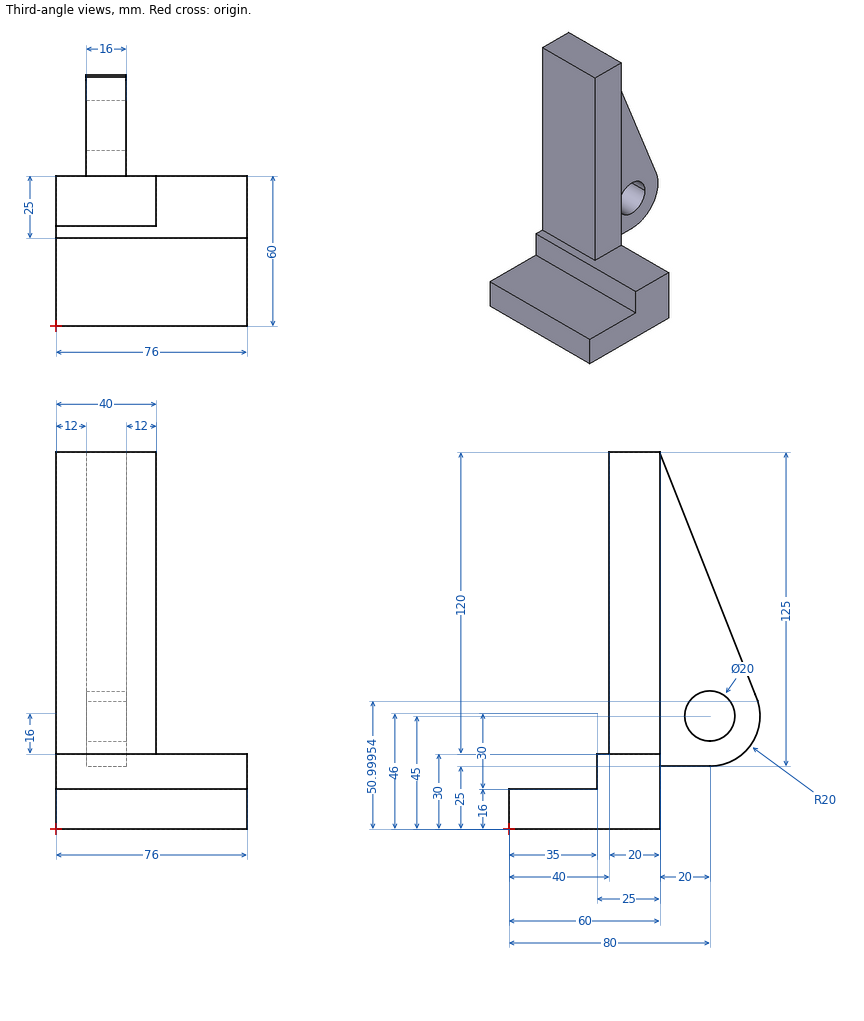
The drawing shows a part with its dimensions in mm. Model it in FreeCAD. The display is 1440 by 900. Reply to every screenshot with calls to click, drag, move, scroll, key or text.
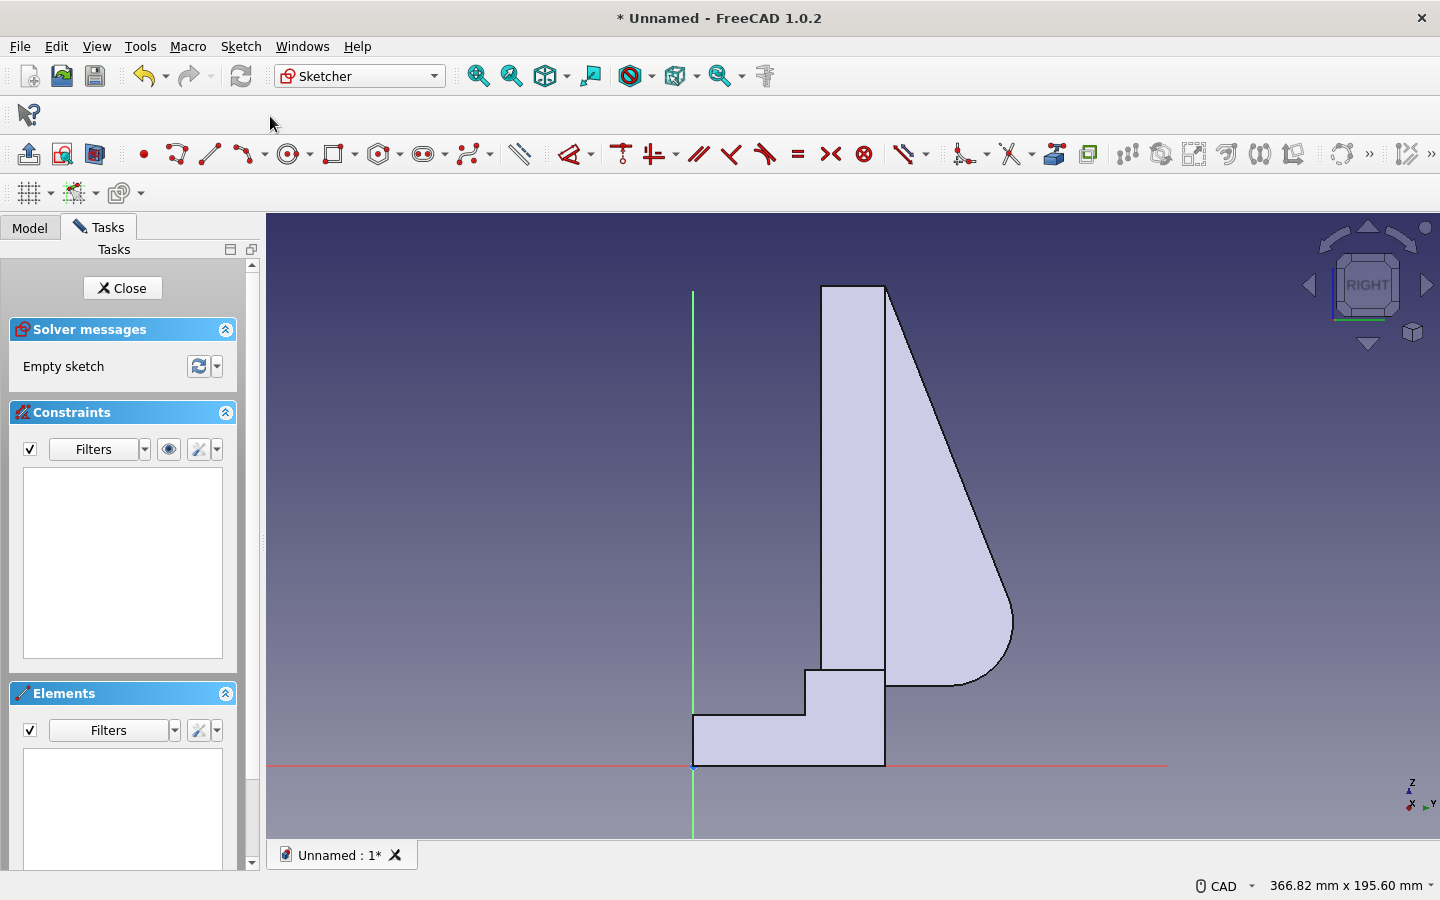
scroll(982, 641, up, 9)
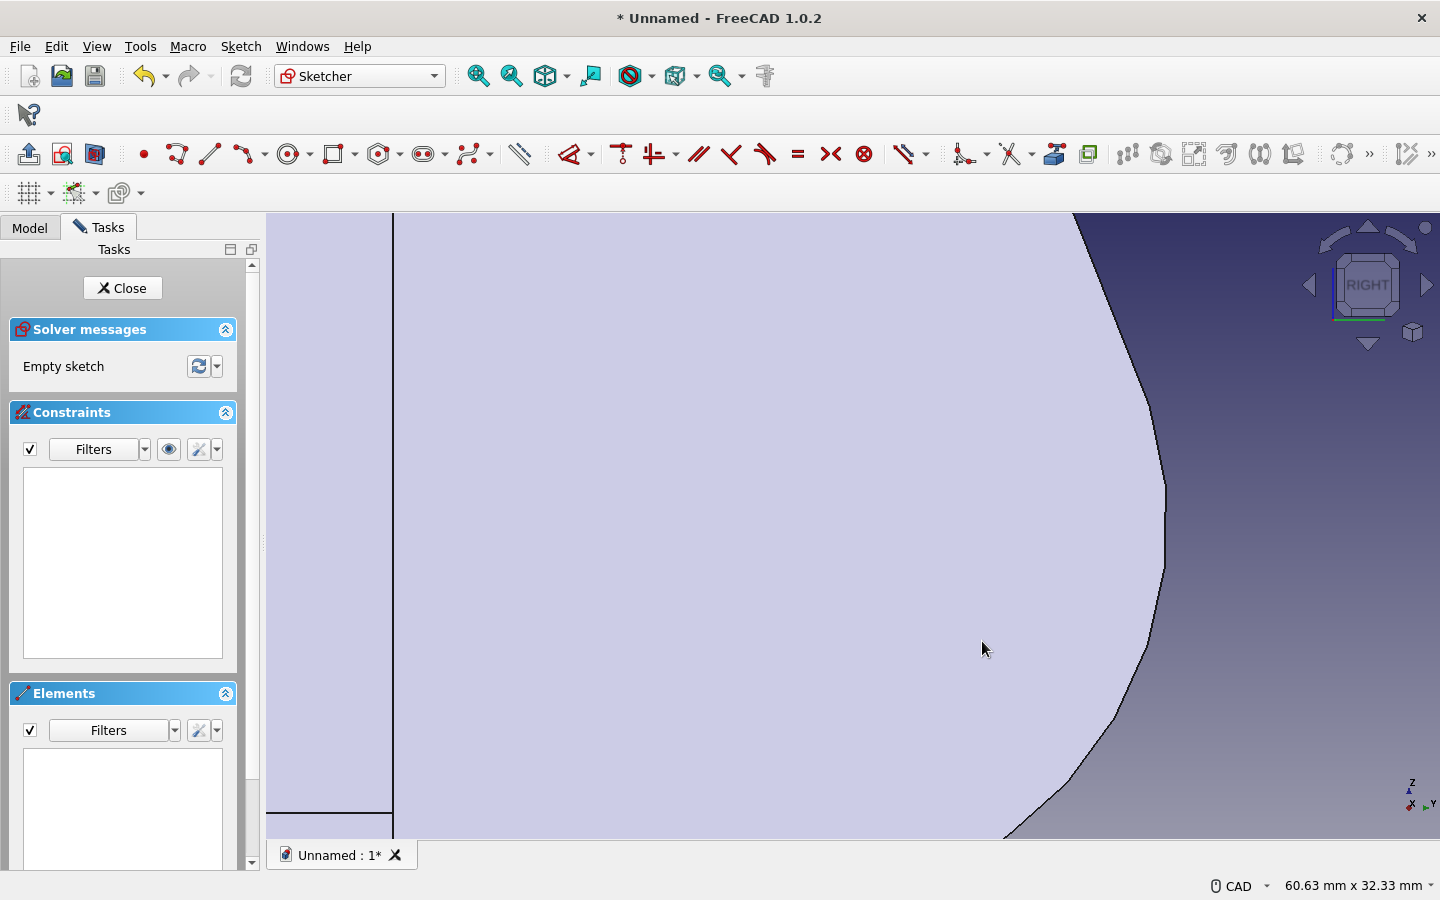
key(g)
key(c)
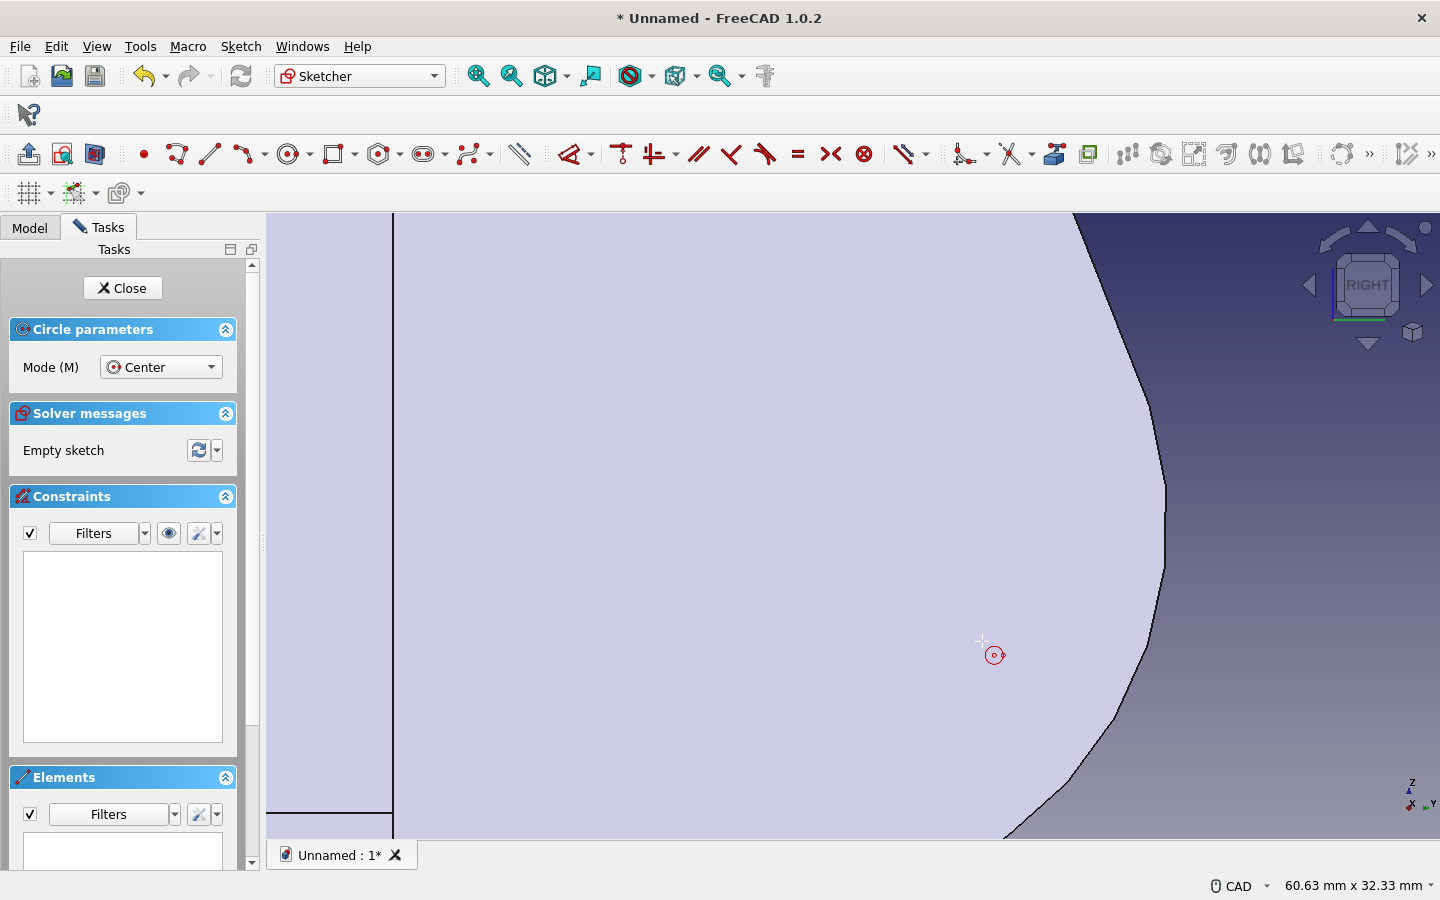
click(780, 523)
click(917, 386)
key(Escape)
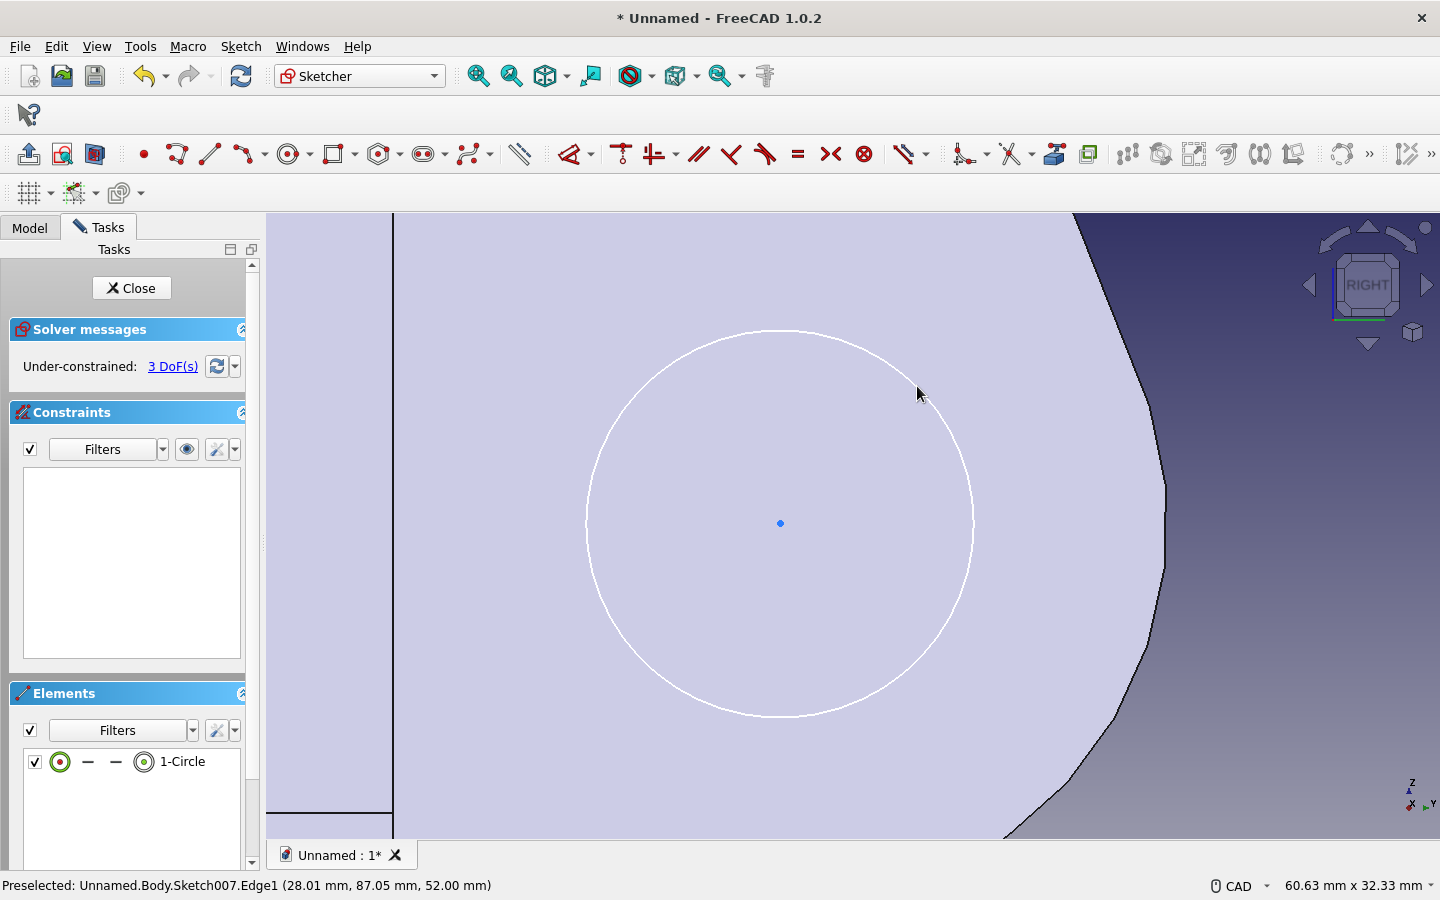
key(d)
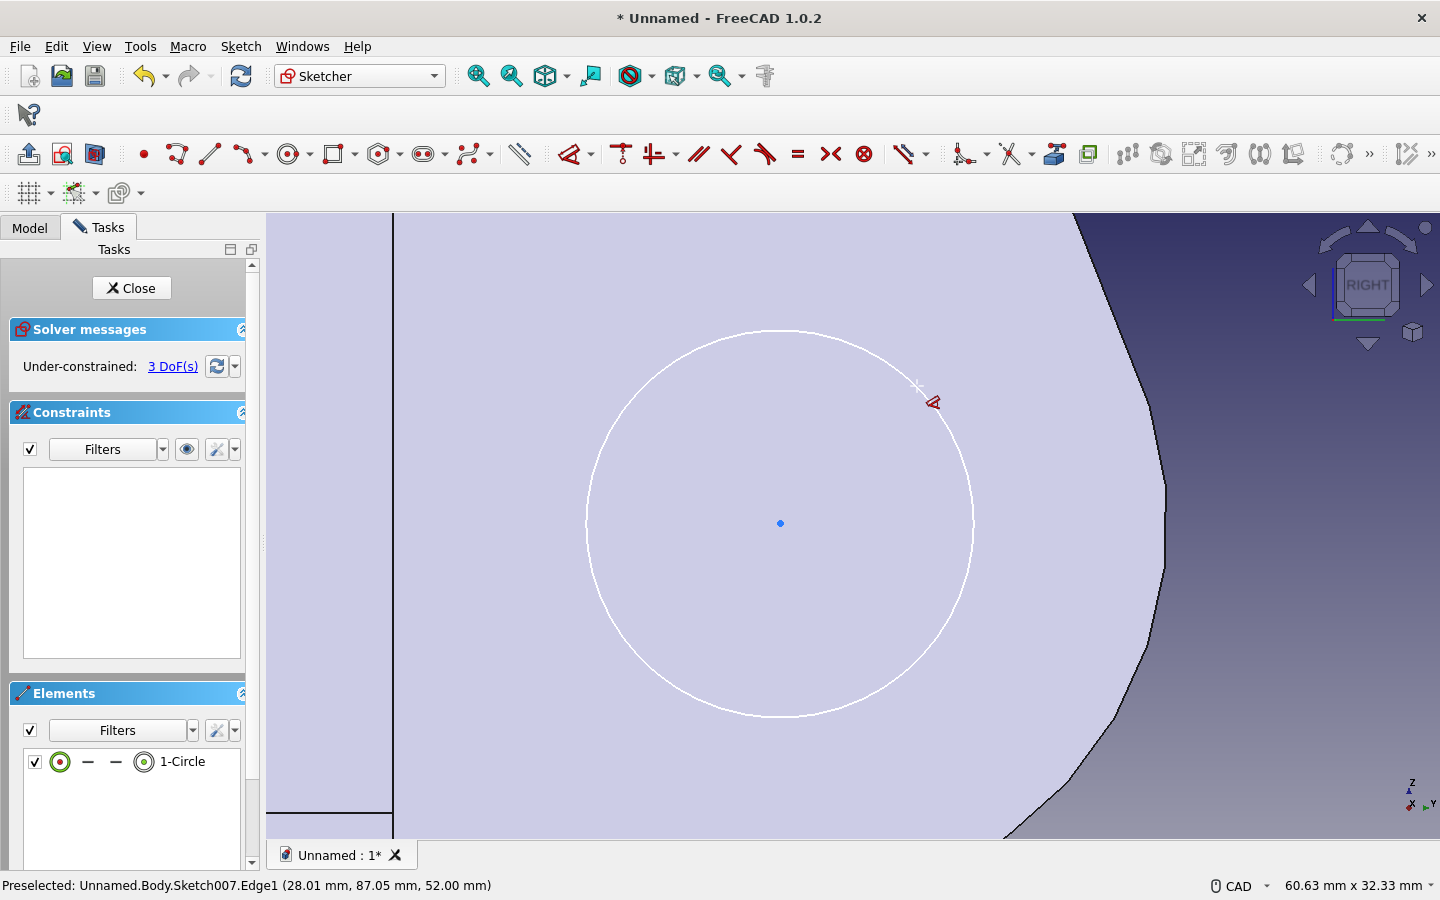
click(917, 387)
click(940, 364)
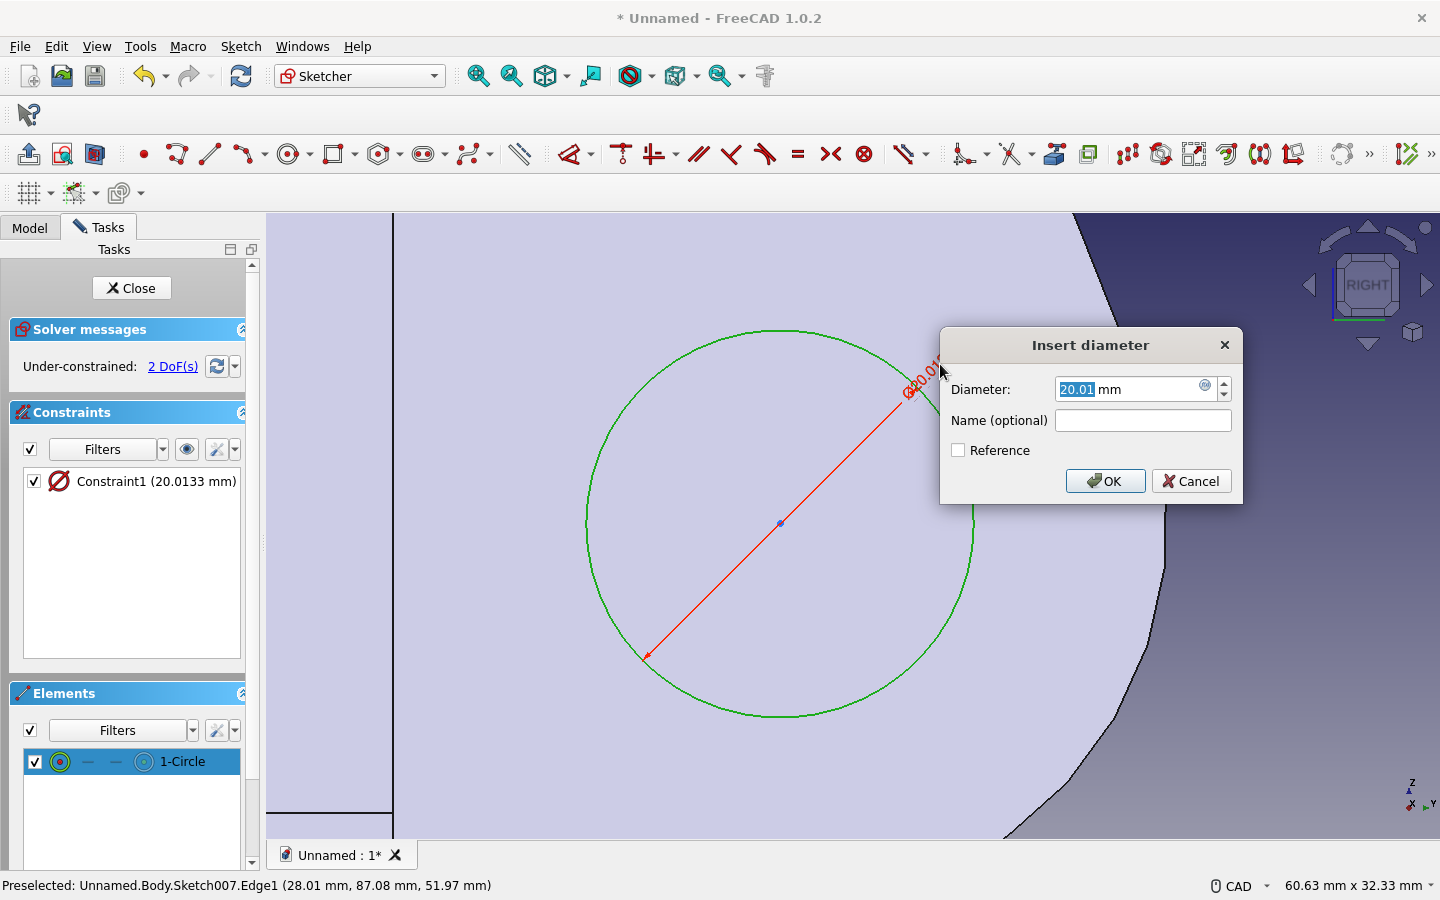
text(20)
key(Return)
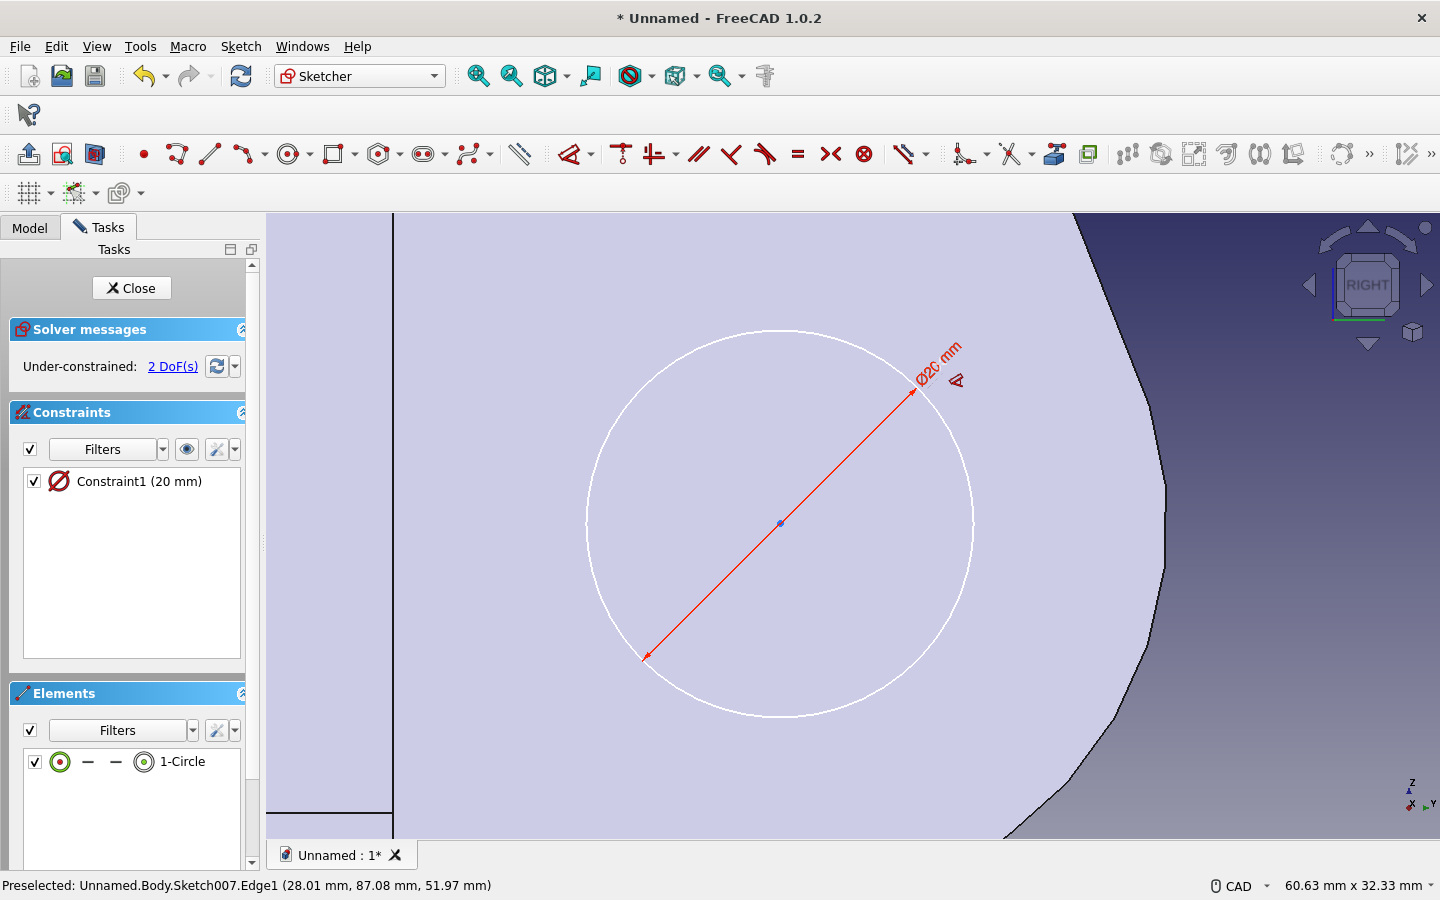
click(780, 524)
click(537, 490)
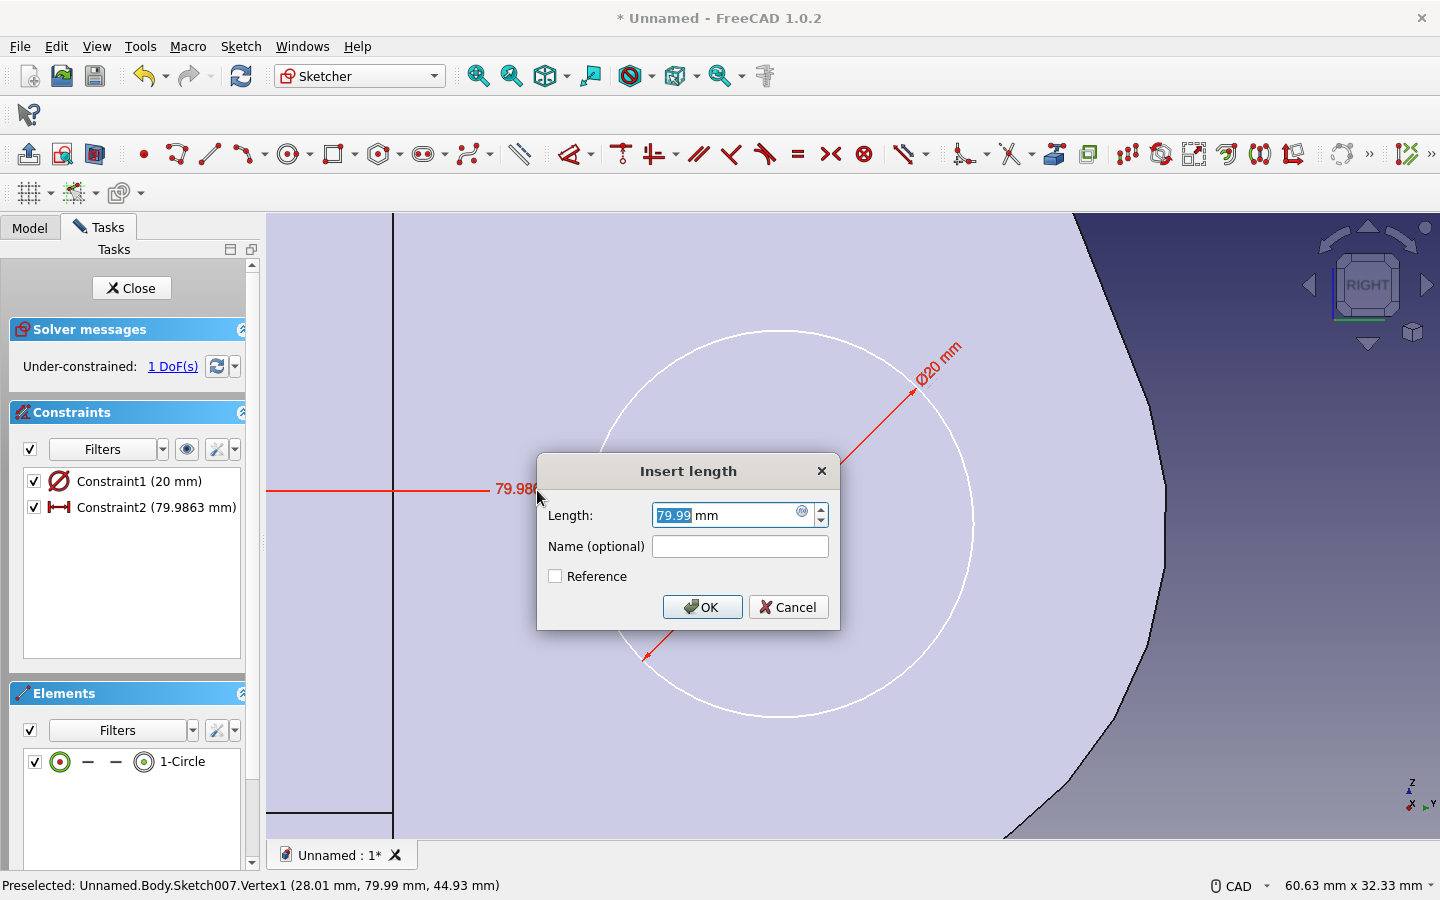
text(80)
key(Return)